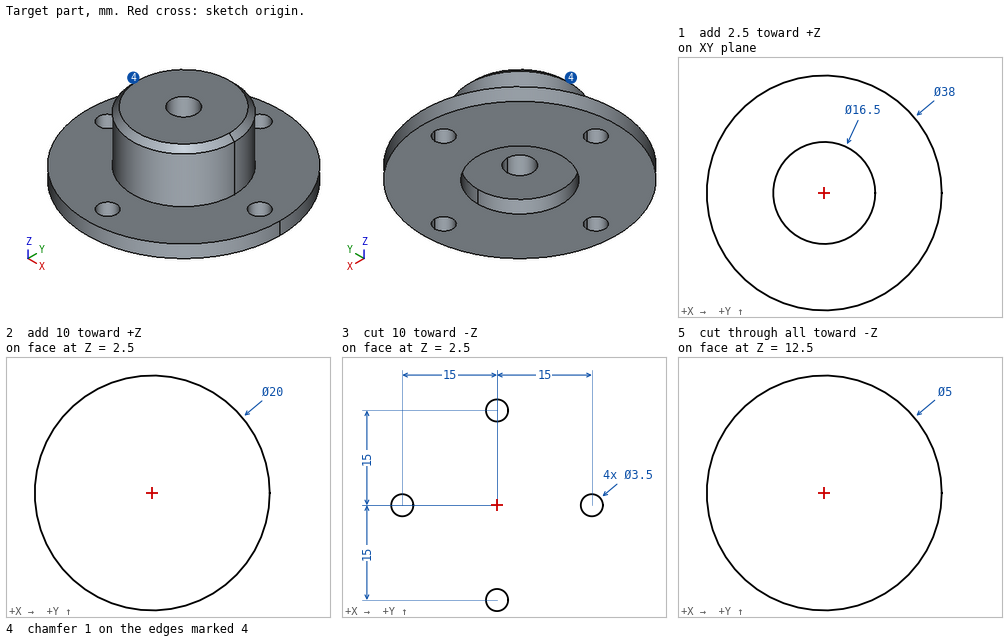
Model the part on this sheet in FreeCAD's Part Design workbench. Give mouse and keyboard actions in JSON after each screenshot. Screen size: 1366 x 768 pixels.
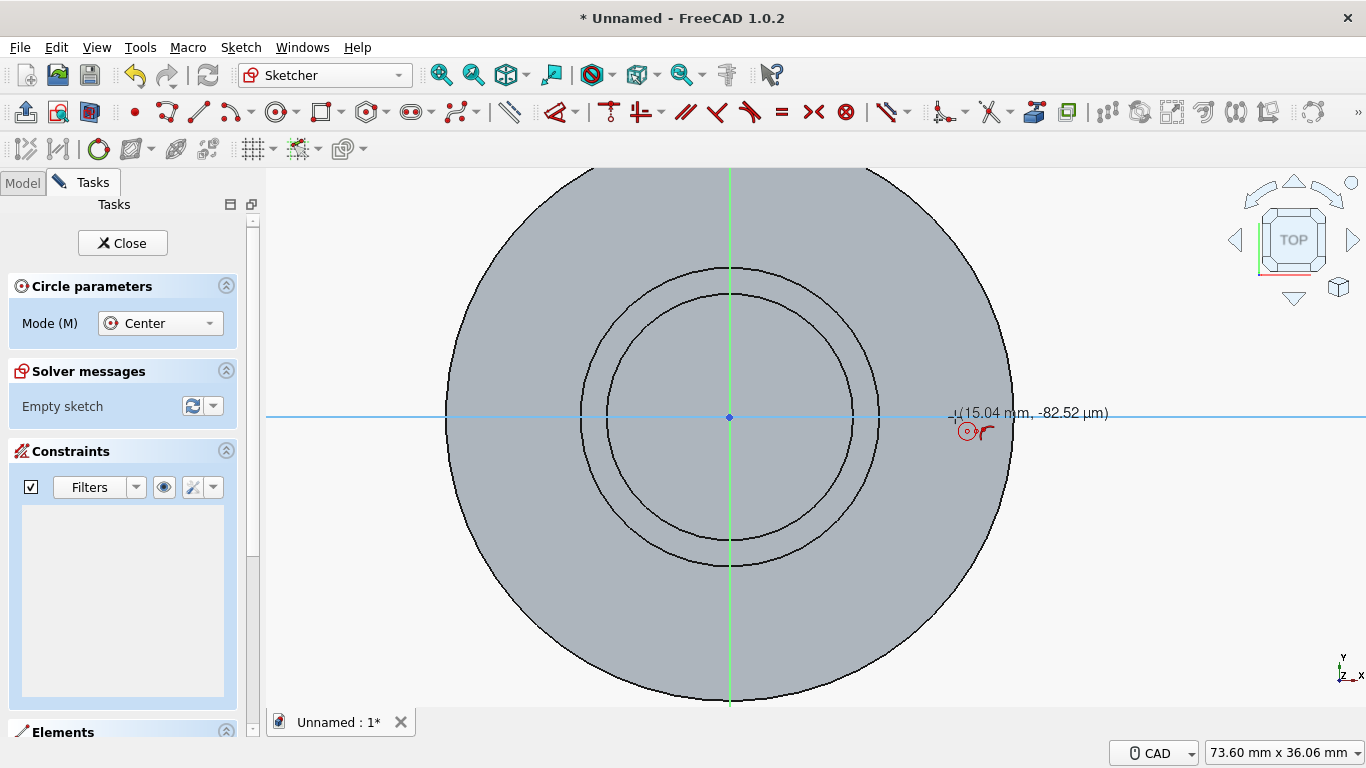
{"action": "left_click", "coordinate": [954, 417]}
{"action": "mouse_move", "coordinate": [973, 399]}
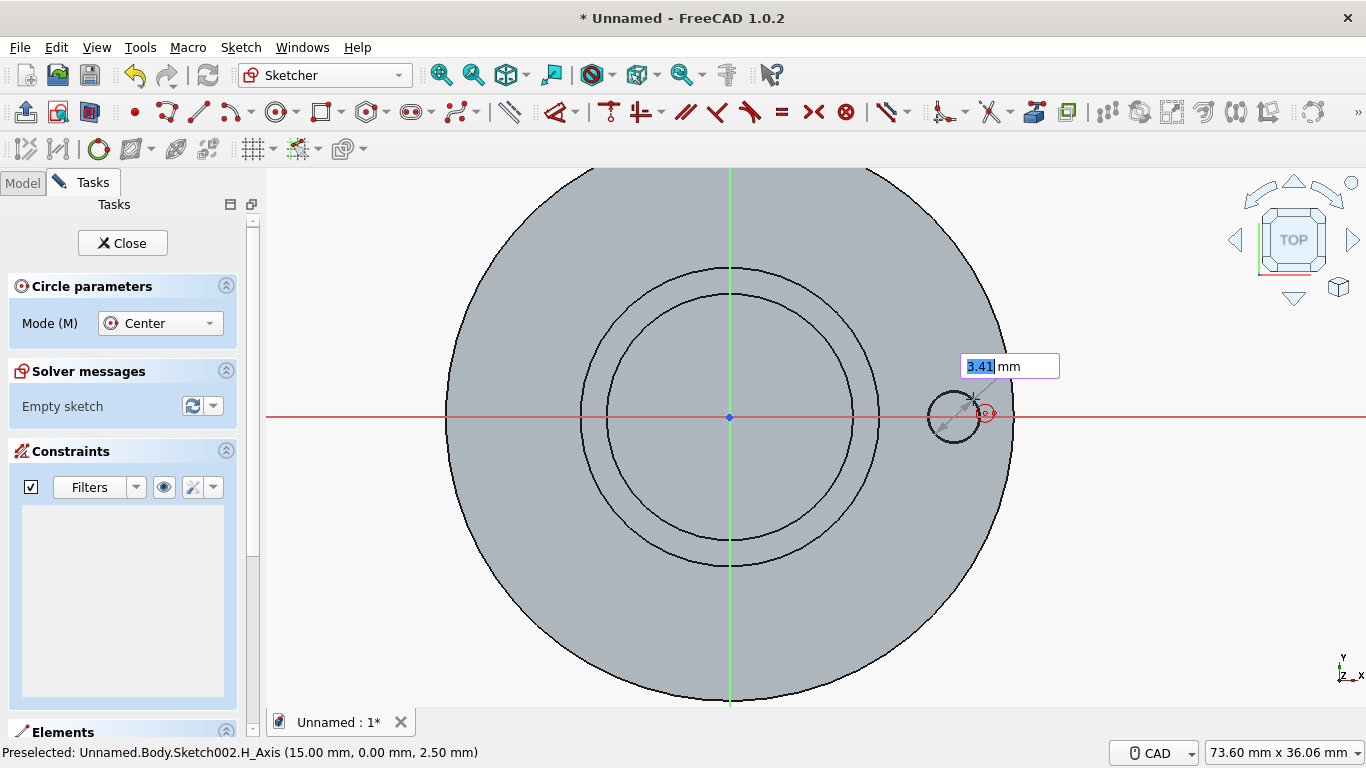
{"action": "type", "text": "3.5"}
{"action": "key", "text": "Return"}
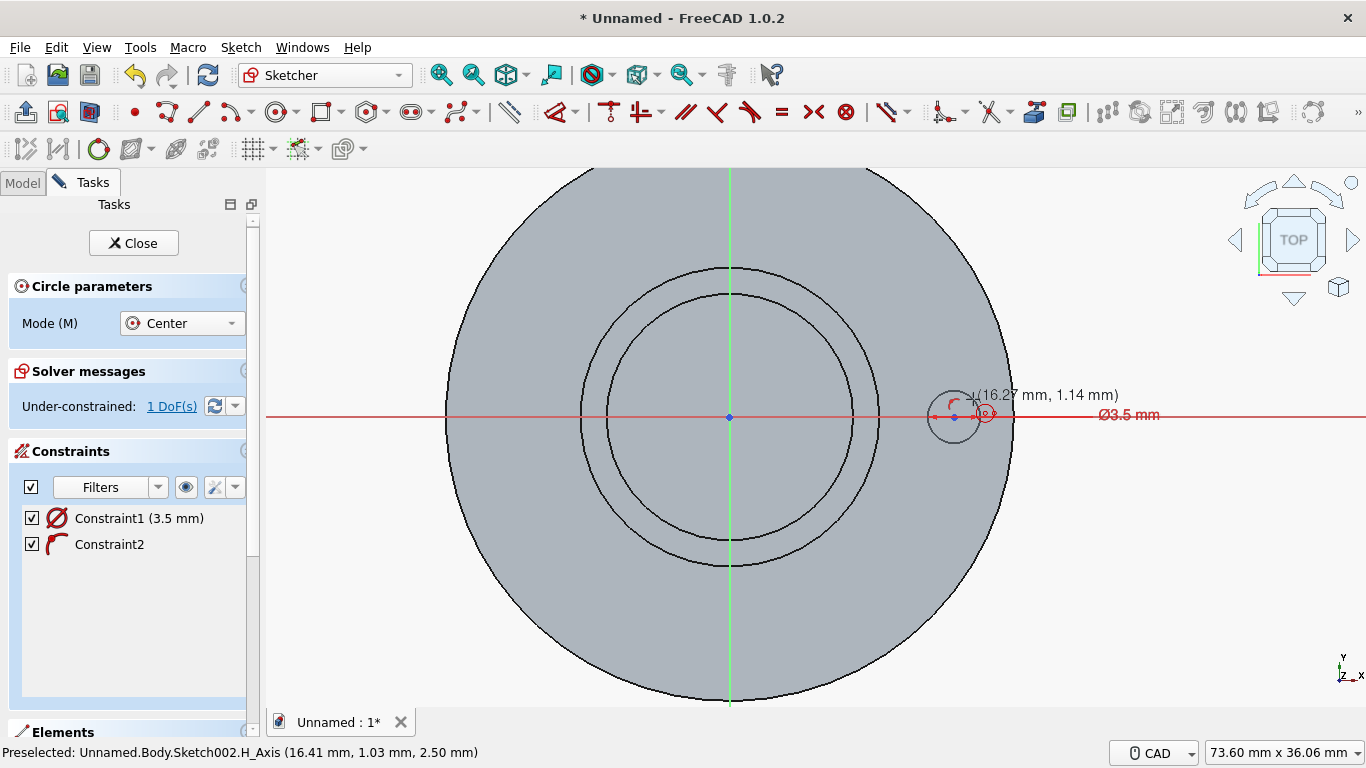
{"action": "scroll", "coordinate": [783, 479], "scroll_direction": "down", "scroll_amount": 2}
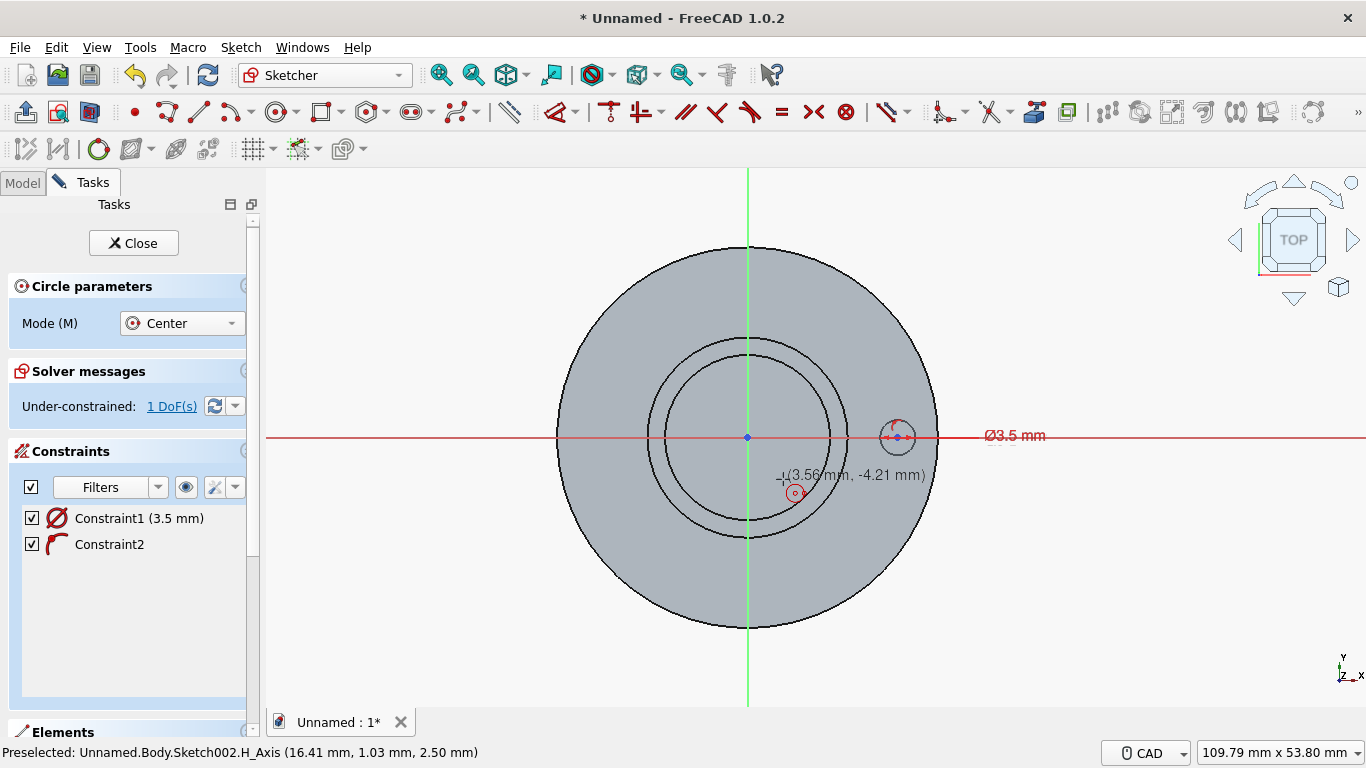
{"action": "scroll", "coordinate": [748, 287], "scroll_direction": "up", "scroll_amount": 2}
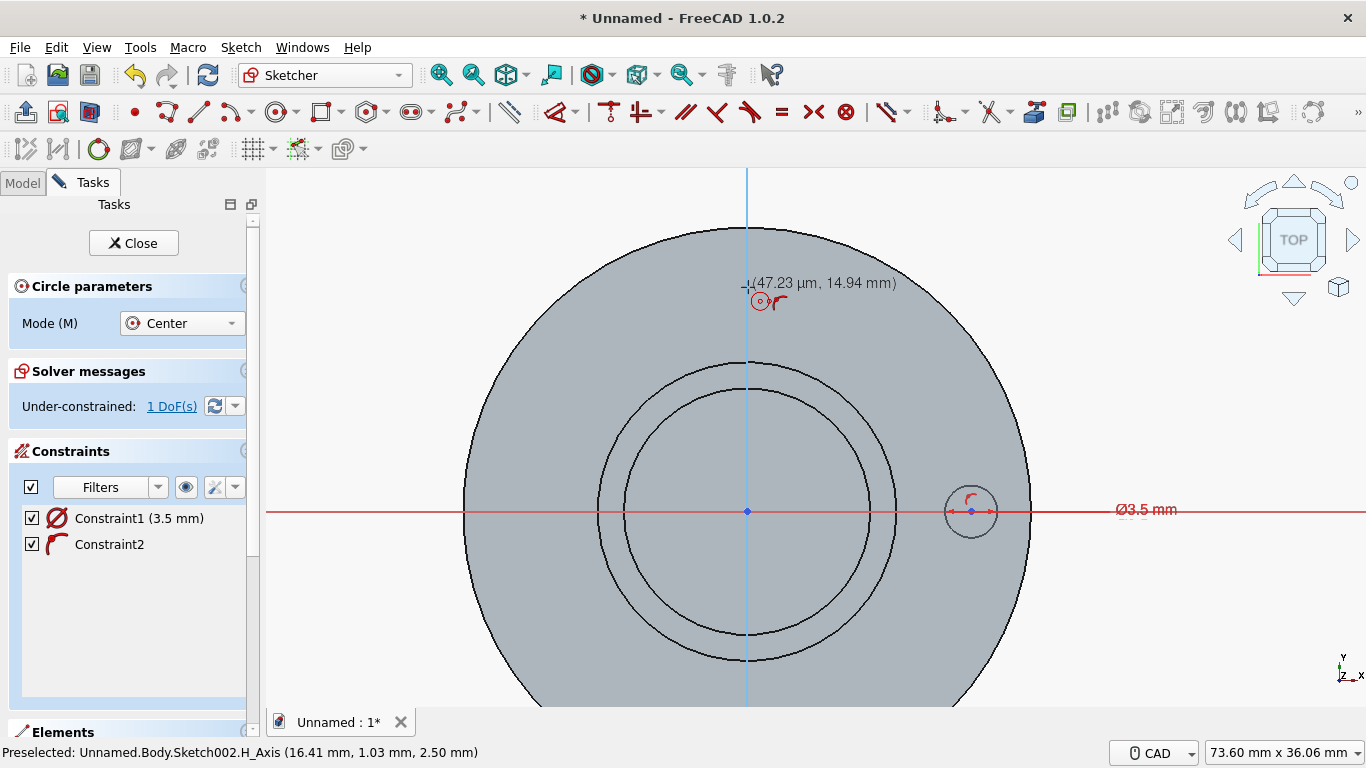
{"action": "left_click", "coordinate": [747, 287]}
{"action": "mouse_move", "coordinate": [766, 269]}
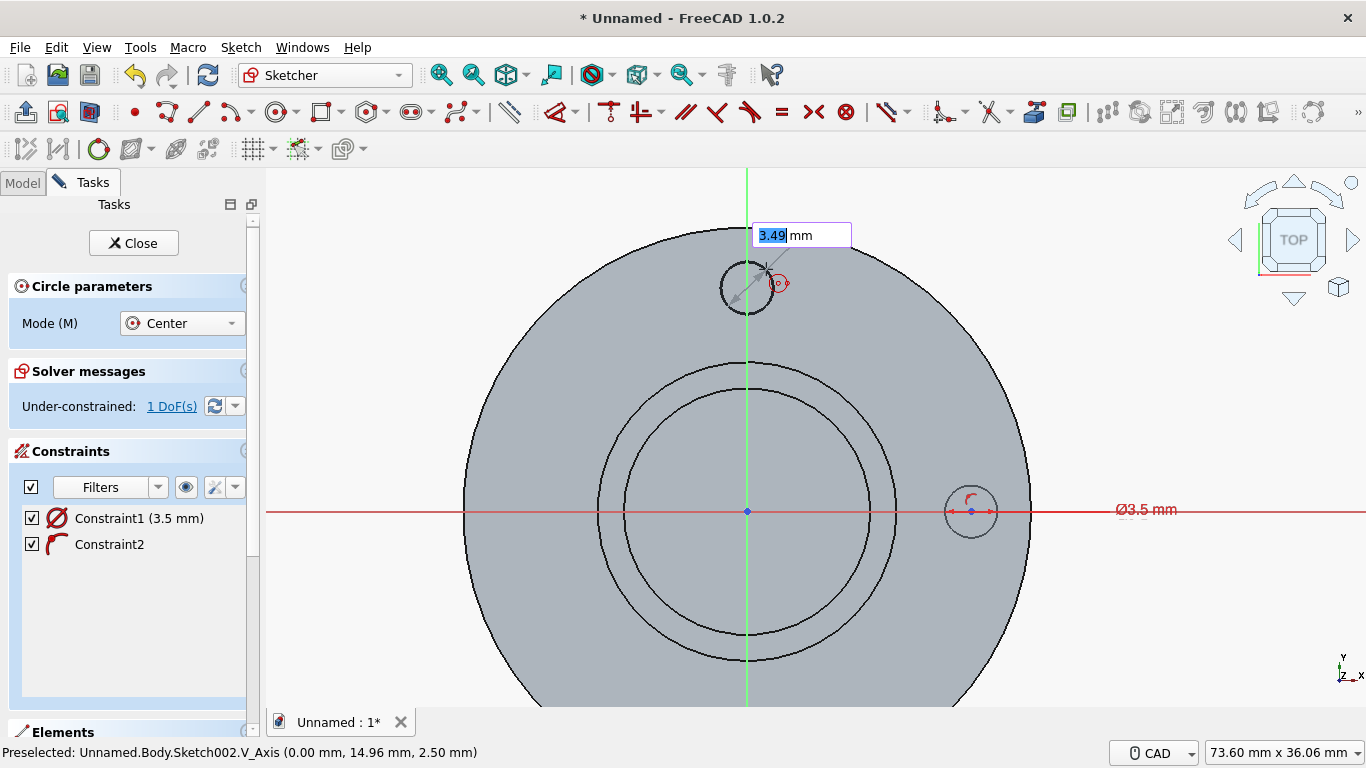
{"action": "type", "text": "3.5"}
{"action": "key", "text": "Return"}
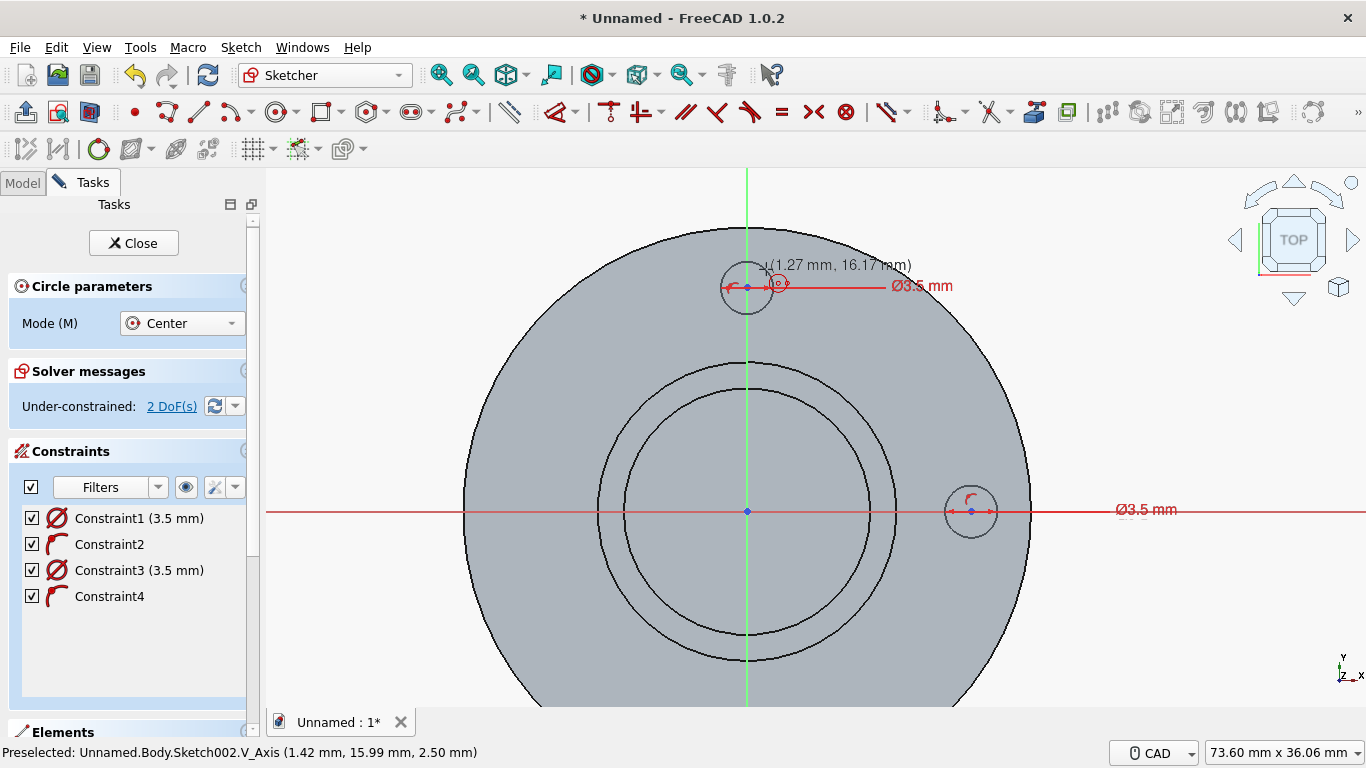
{"action": "left_click", "coordinate": [523, 512]}
{"action": "mouse_move", "coordinate": [541, 493]}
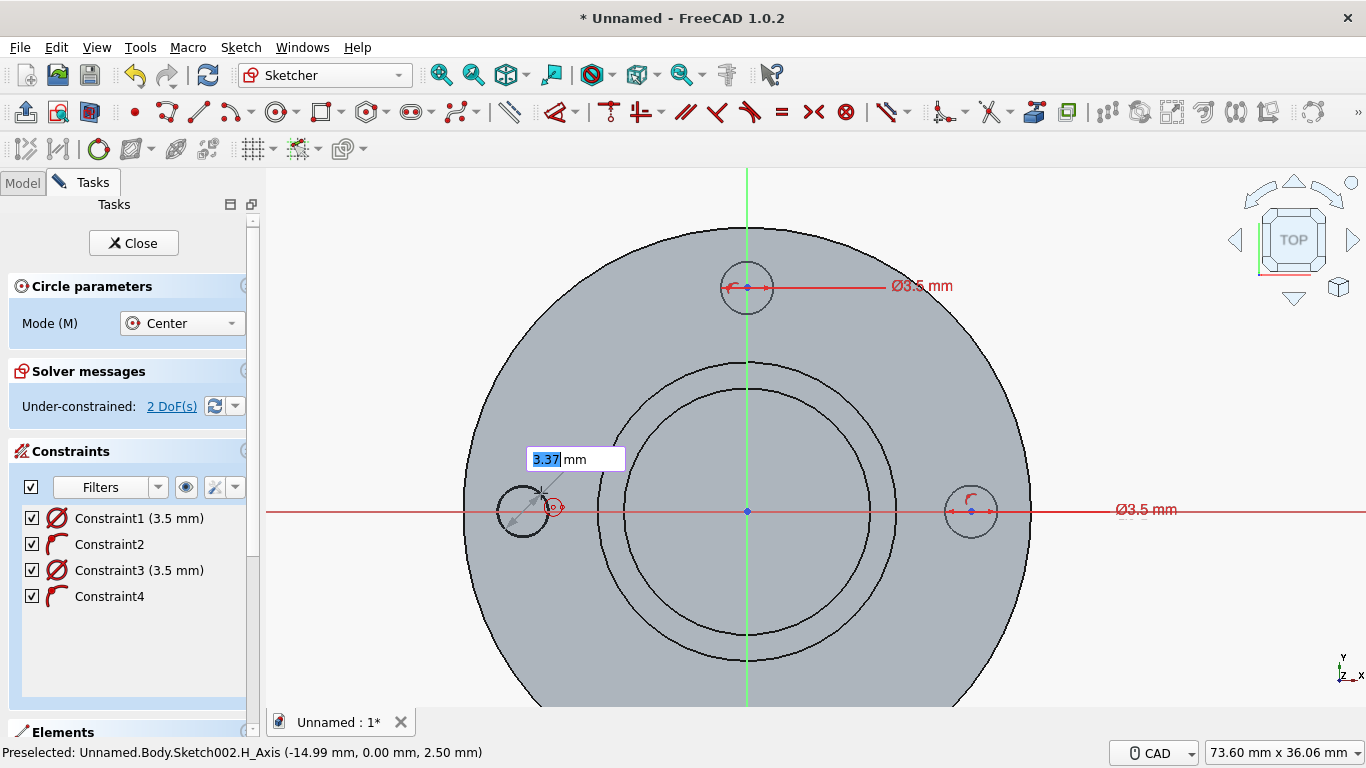
{"action": "type", "text": "3.5"}
{"action": "key", "text": "Return"}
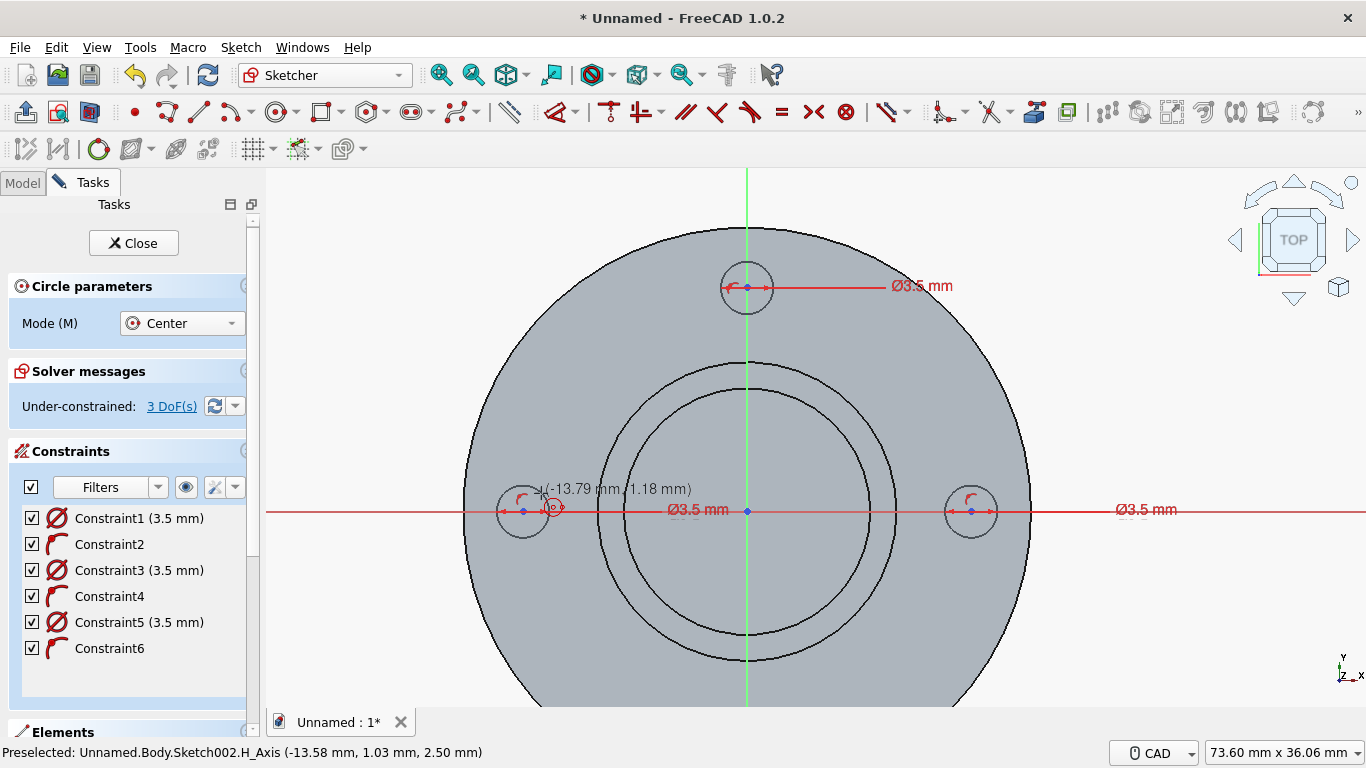
{"action": "scroll", "coordinate": [748, 287], "scroll_direction": "down", "scroll_amount": 2}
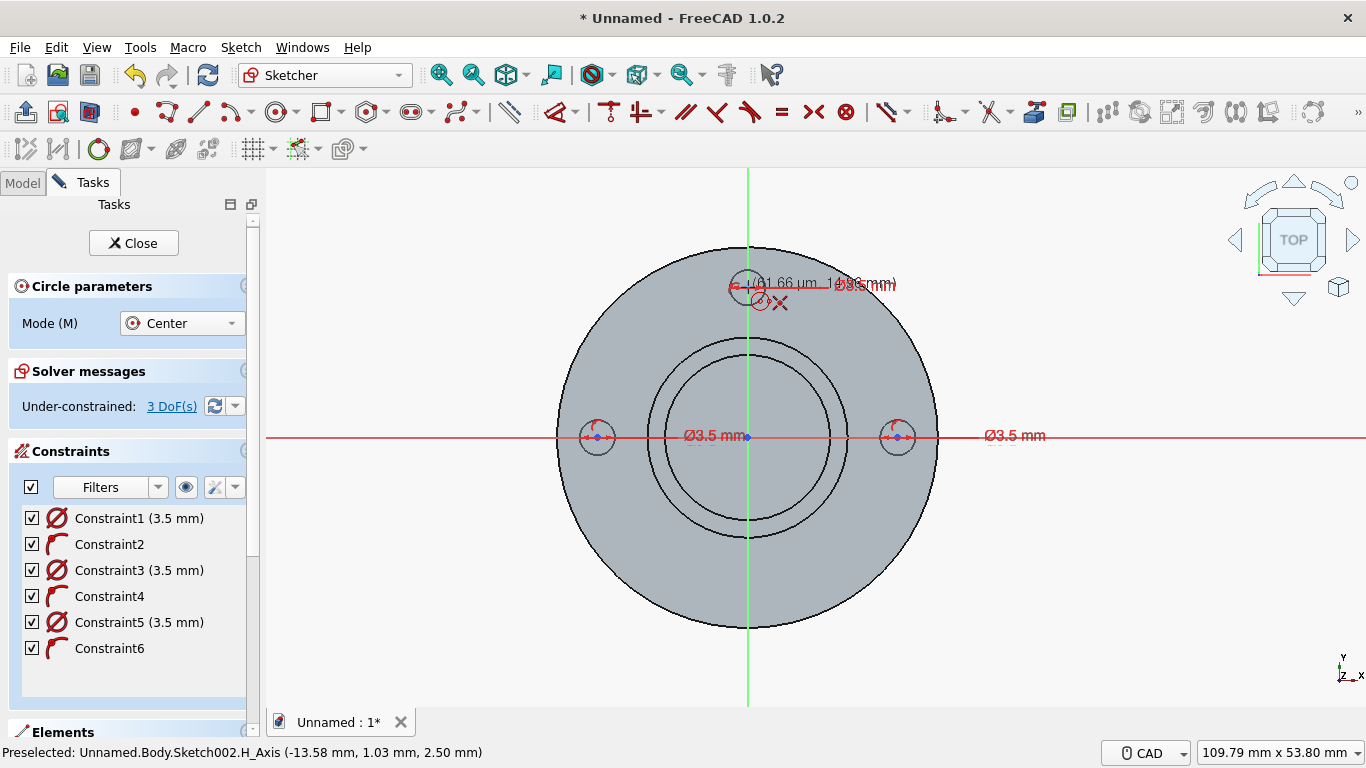
{"action": "scroll", "coordinate": [748, 588], "scroll_direction": "up", "scroll_amount": 2}